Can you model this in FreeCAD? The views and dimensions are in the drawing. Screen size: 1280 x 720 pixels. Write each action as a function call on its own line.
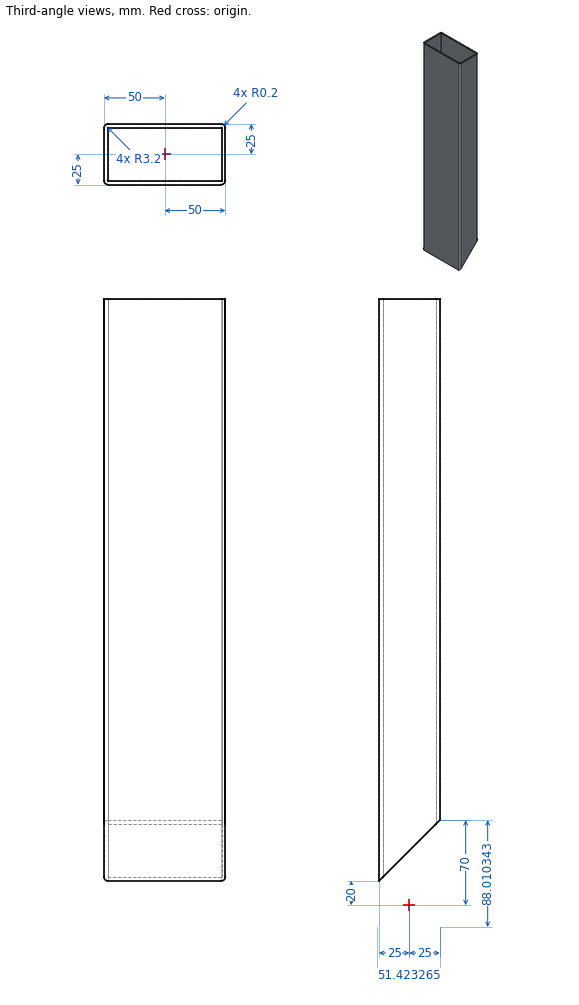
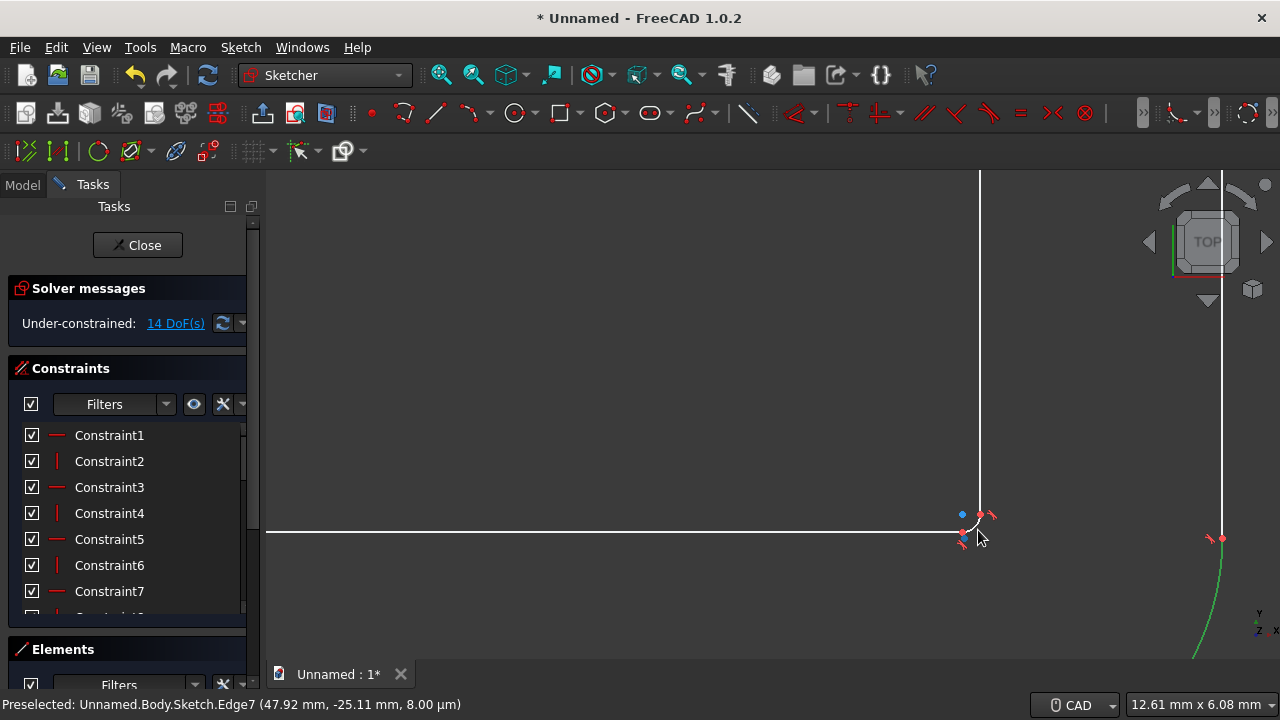
click(975, 527)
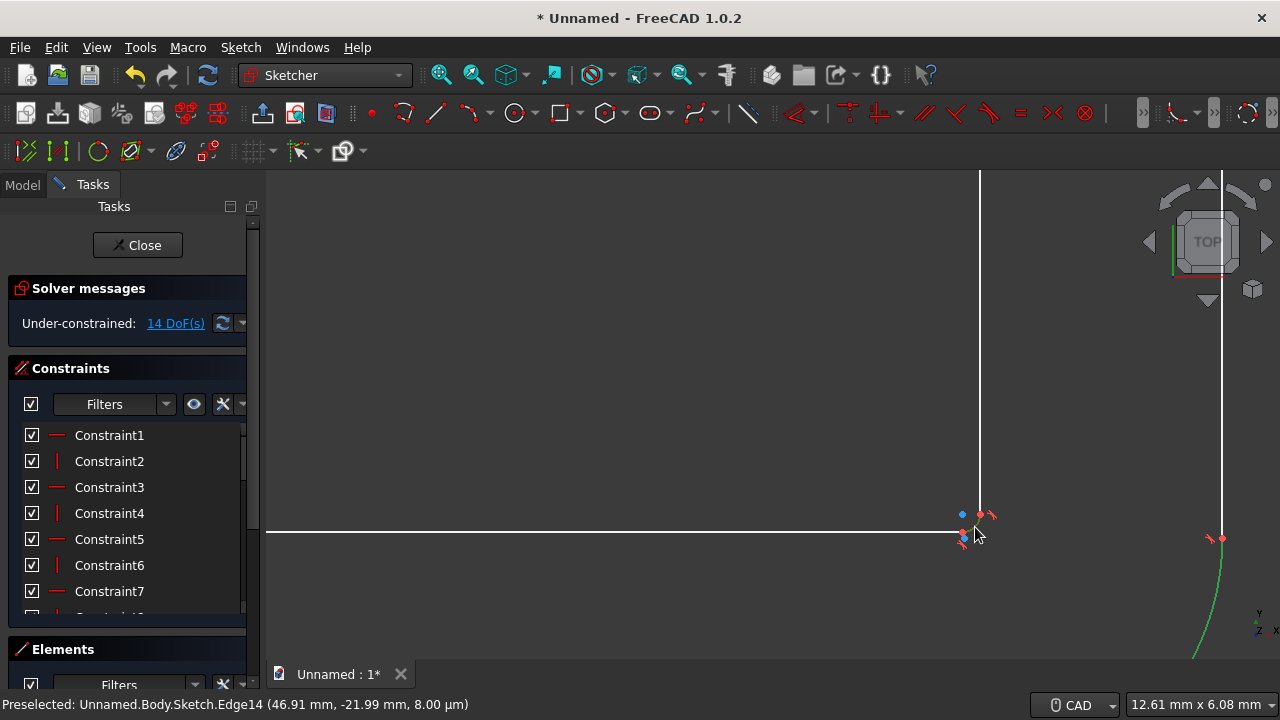
click(848, 114)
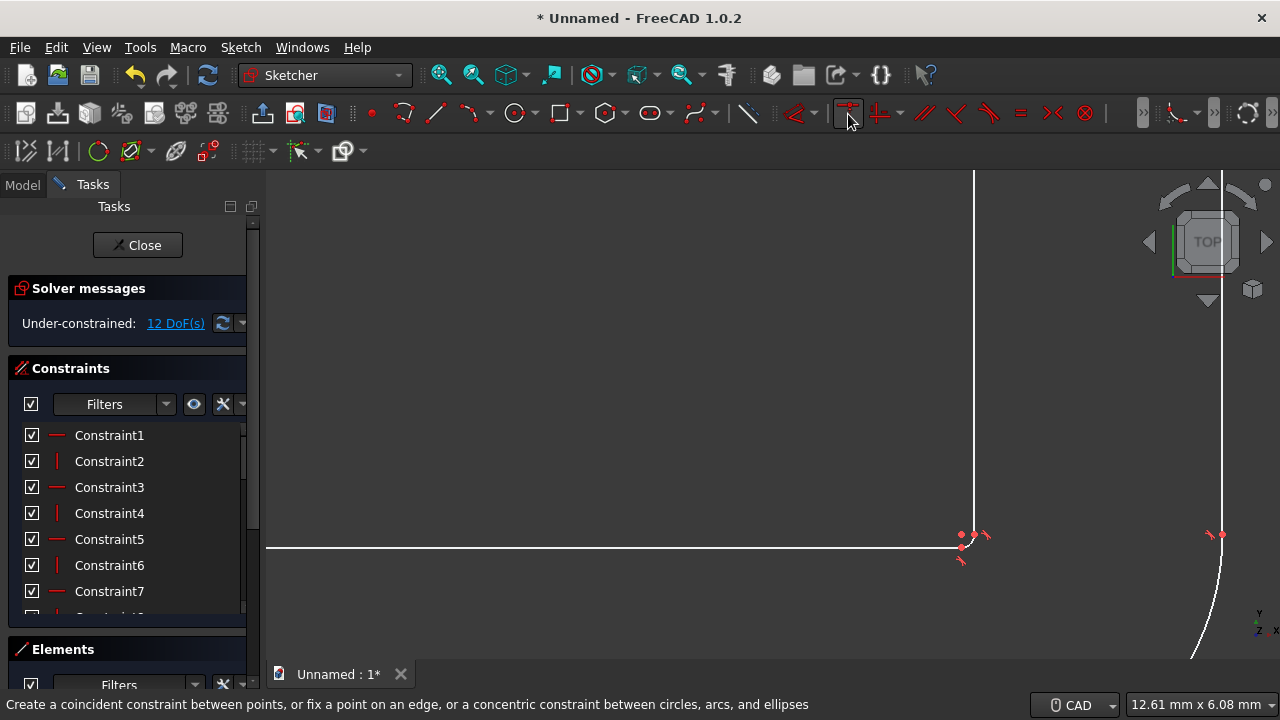
scroll(986, 547, down, 13)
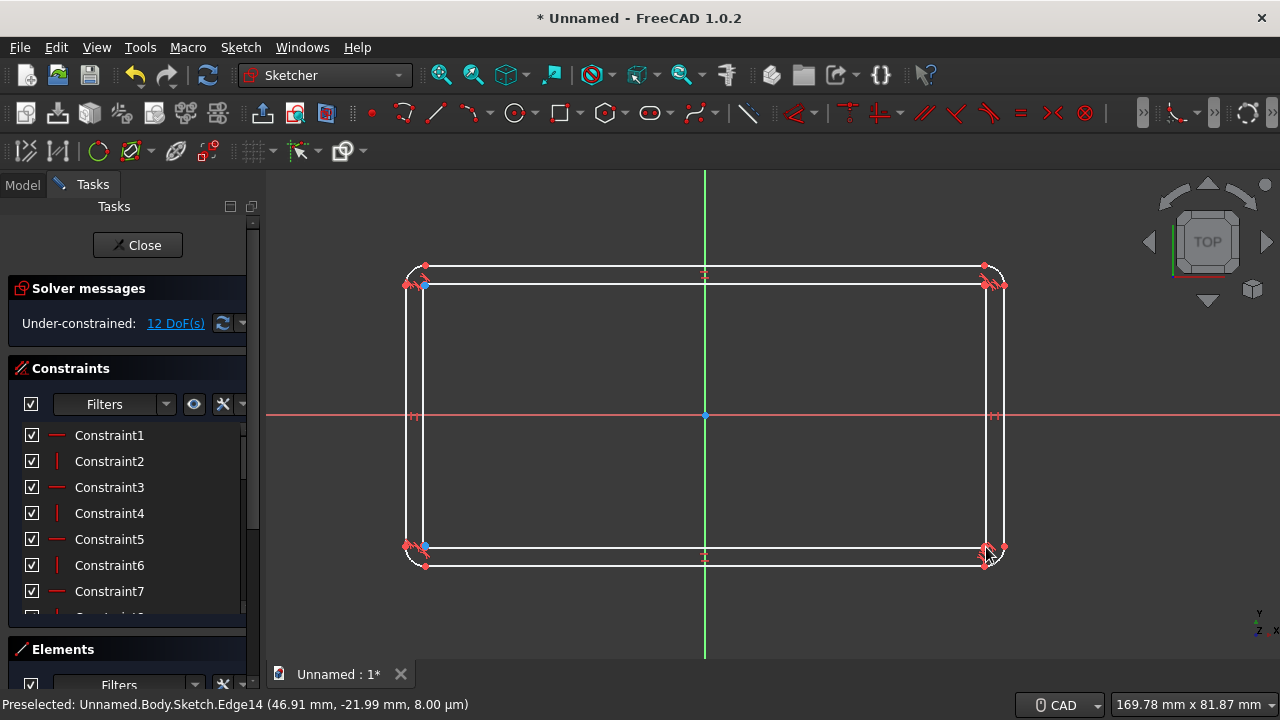
scroll(408, 556, up, 3)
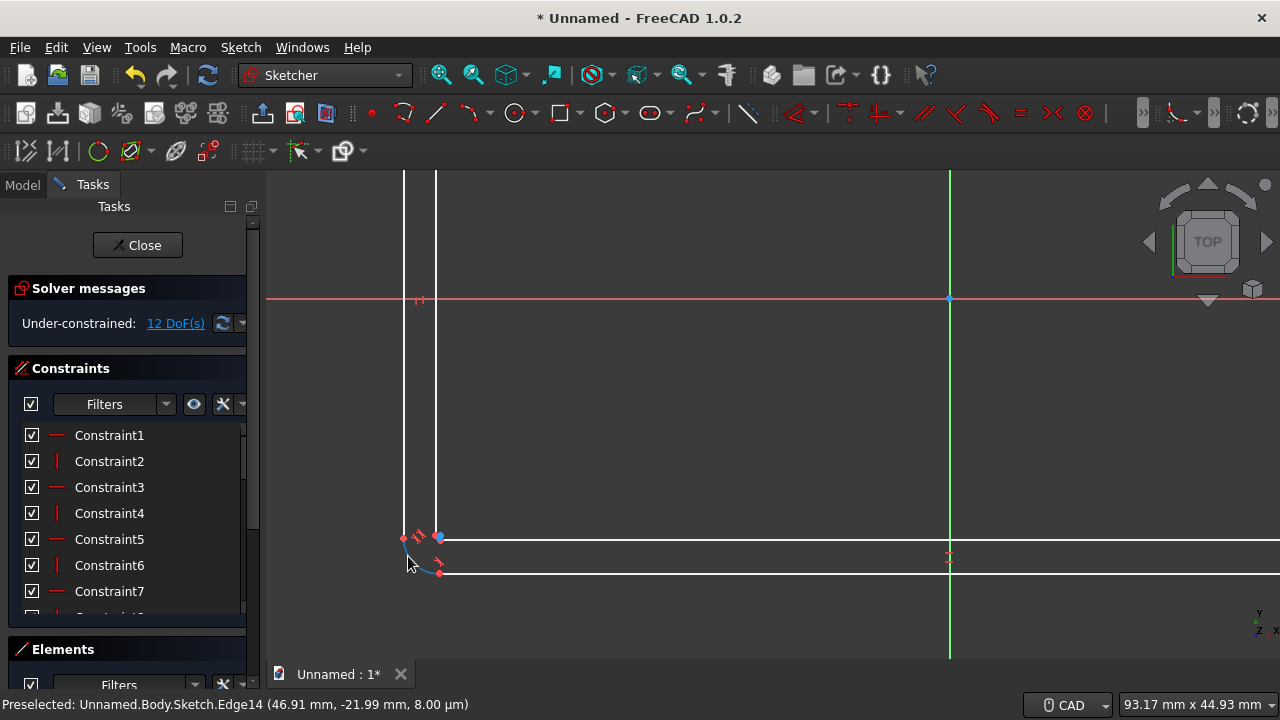
click(408, 555)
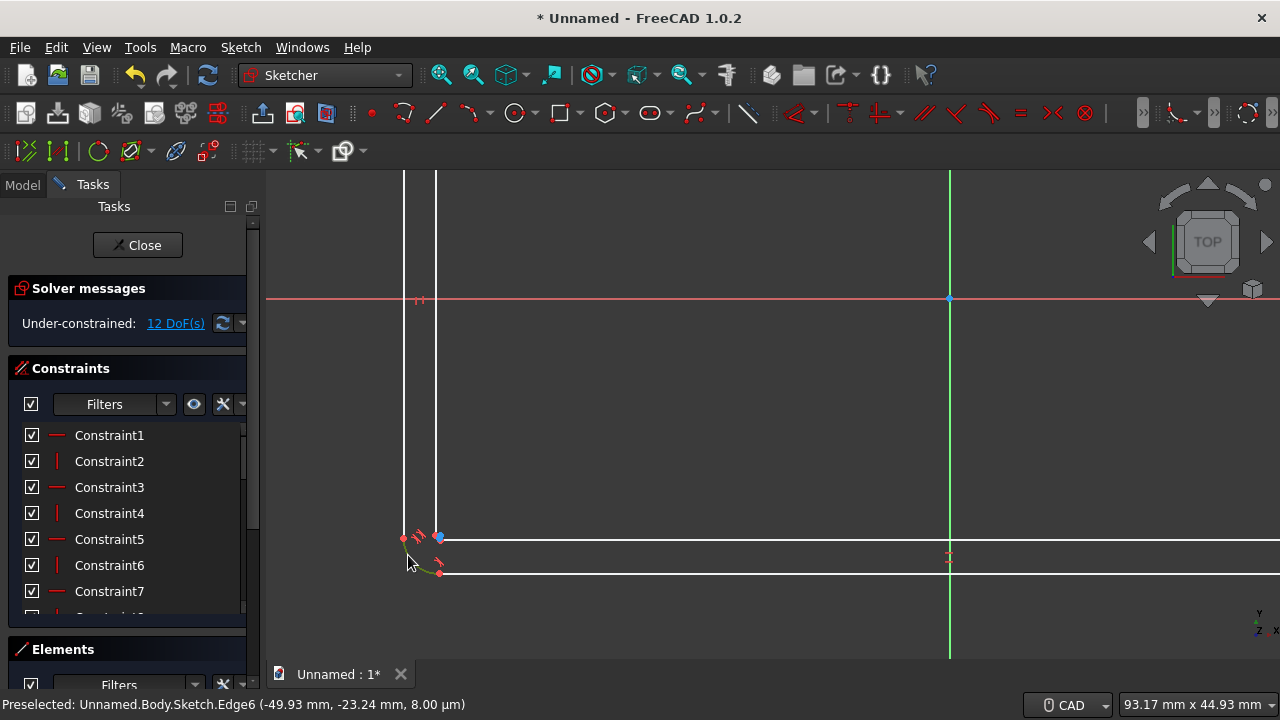
scroll(437, 539, up, 8)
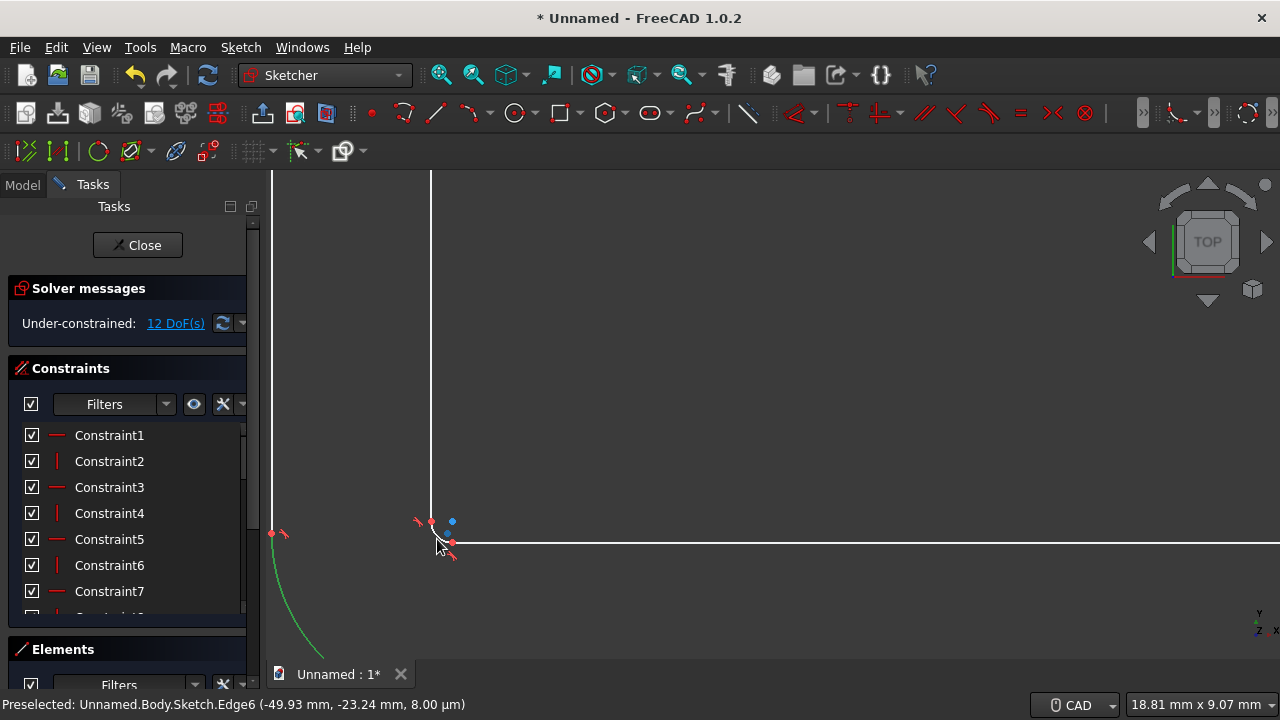
click(437, 536)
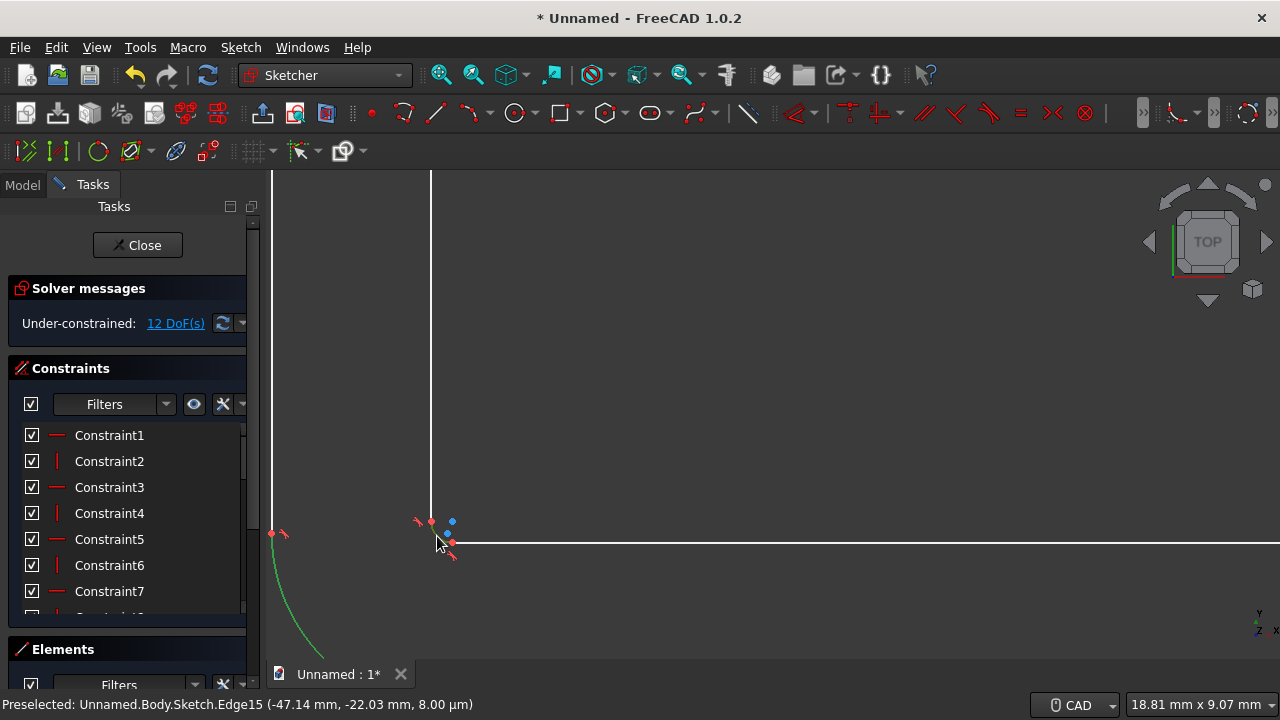
click(848, 114)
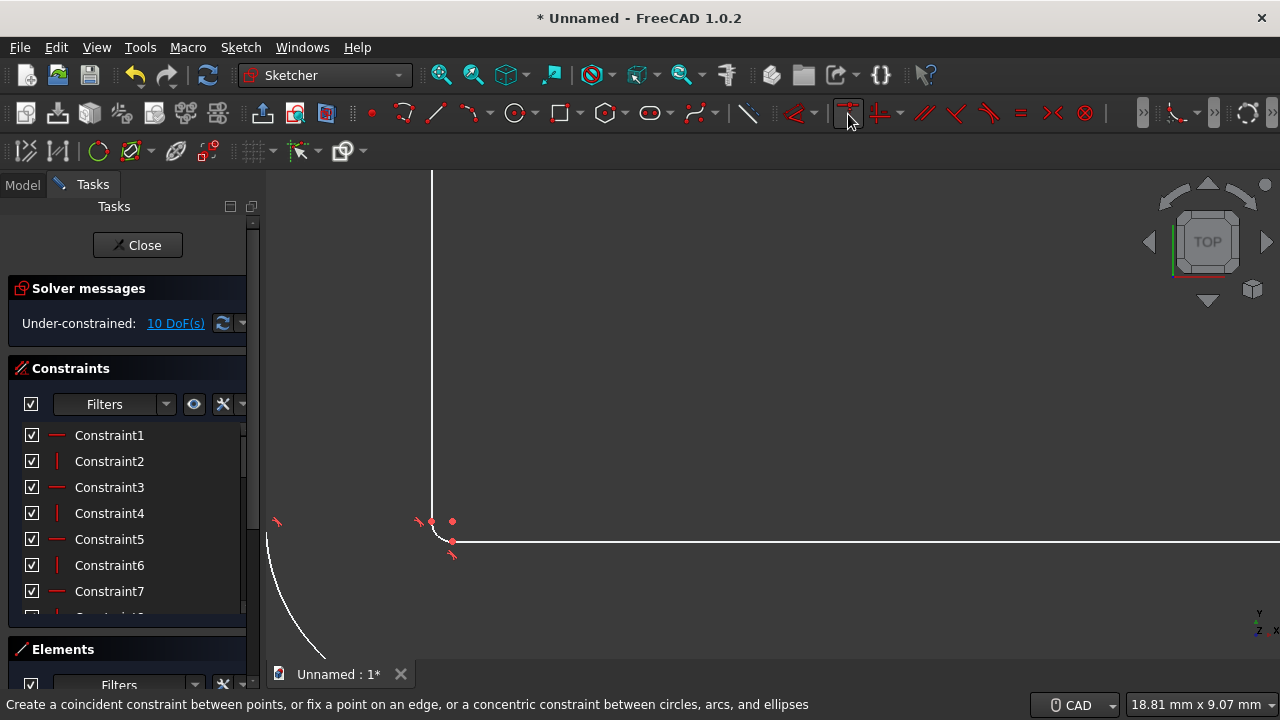
scroll(421, 548, down, 11)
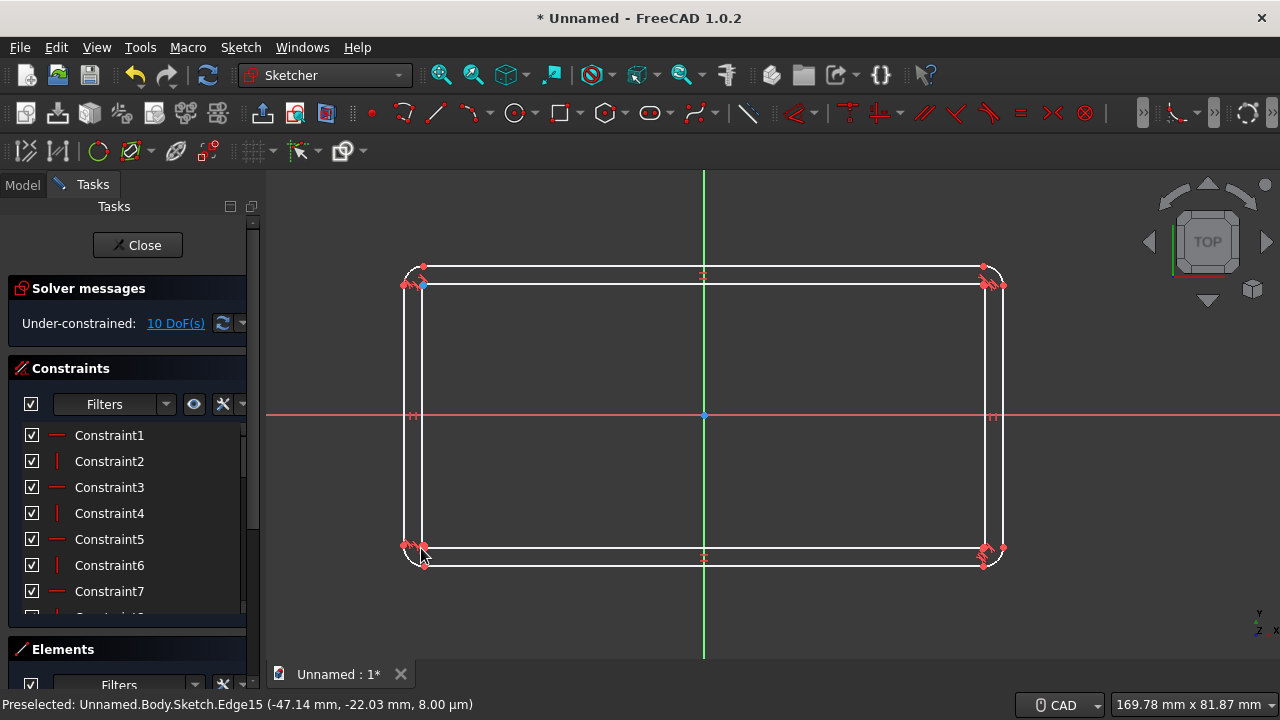
scroll(415, 268, up, 2)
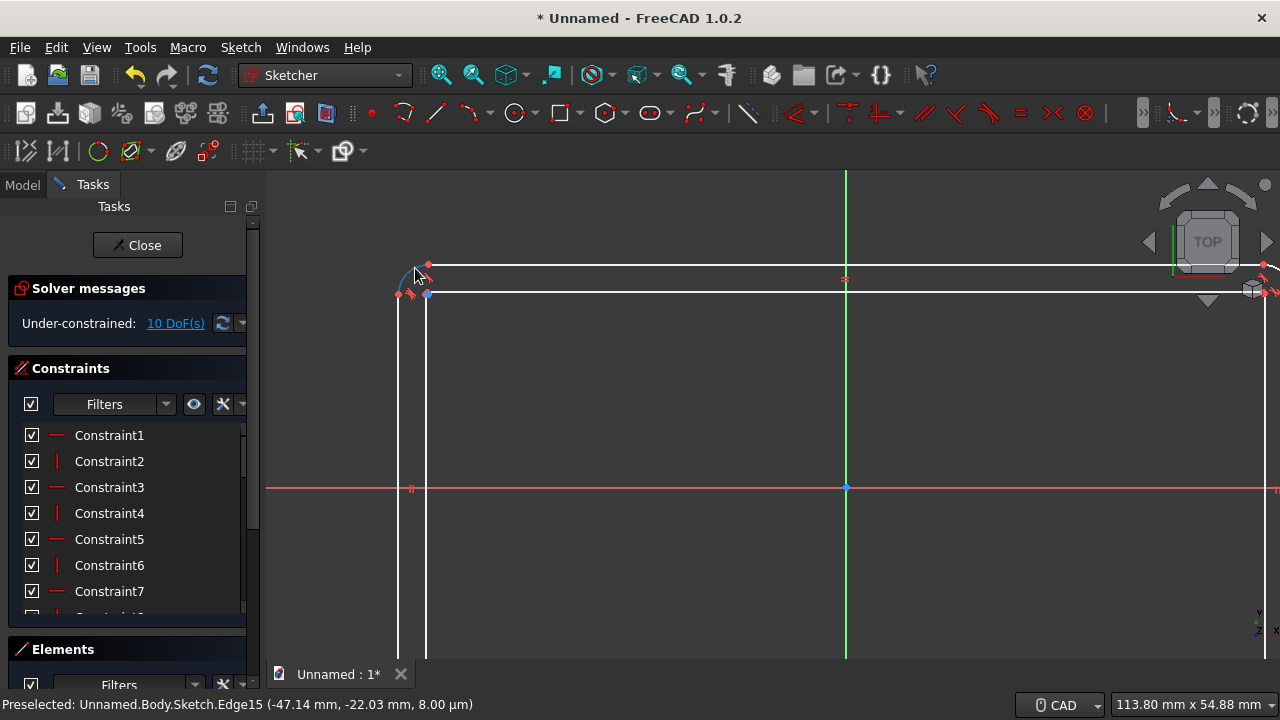
click(415, 268)